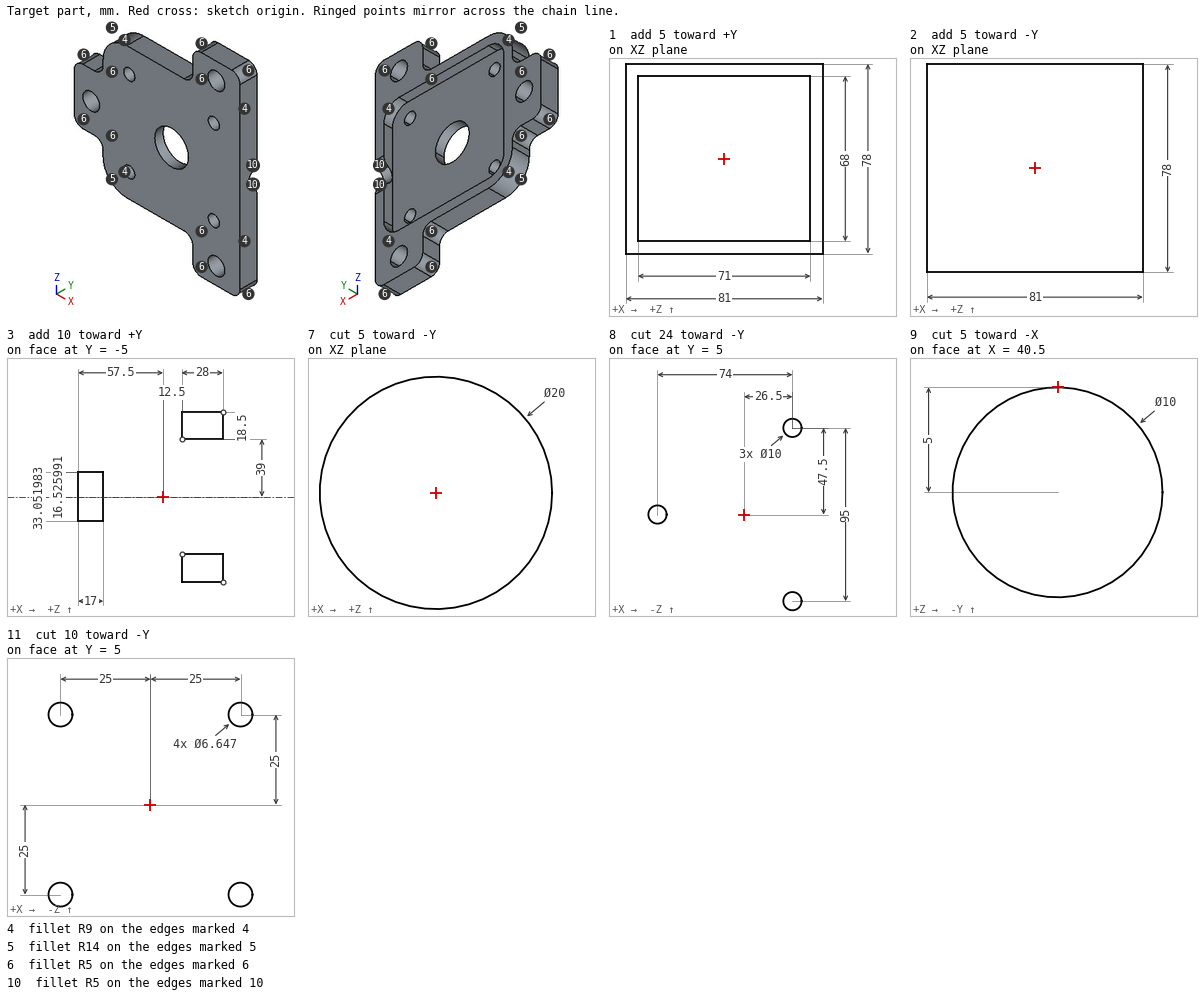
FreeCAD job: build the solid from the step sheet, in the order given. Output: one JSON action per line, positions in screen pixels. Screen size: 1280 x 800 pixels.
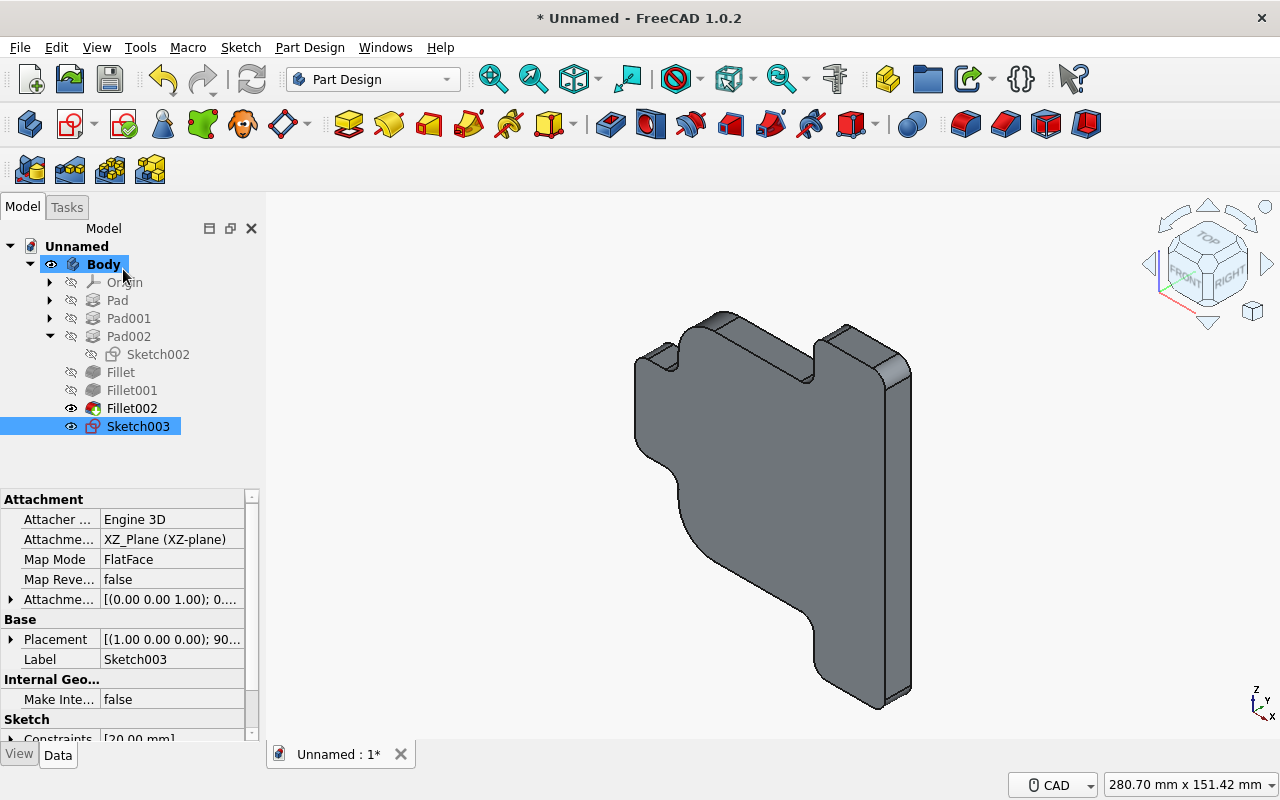
{"action": "left_click", "coordinate": [612, 124]}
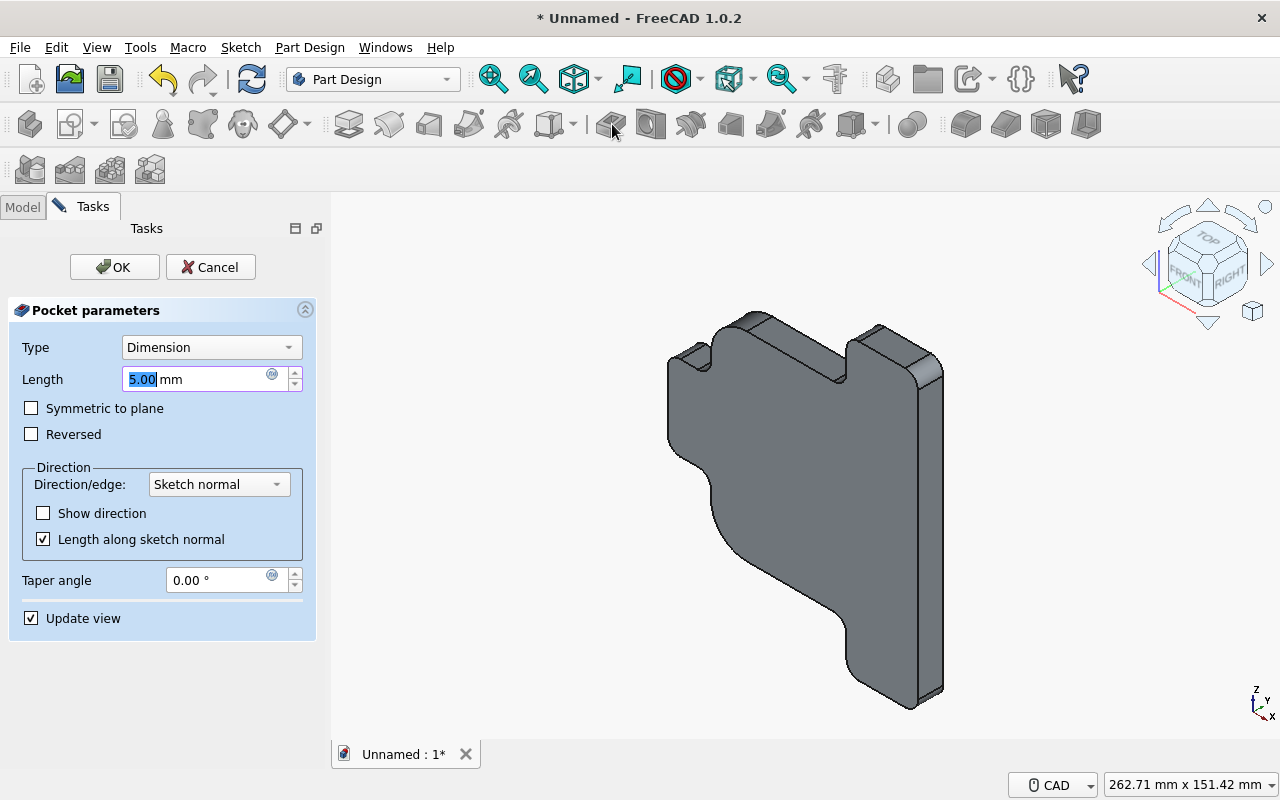
{"action": "type", "text": "5"}
{"action": "key", "text": "Tab"}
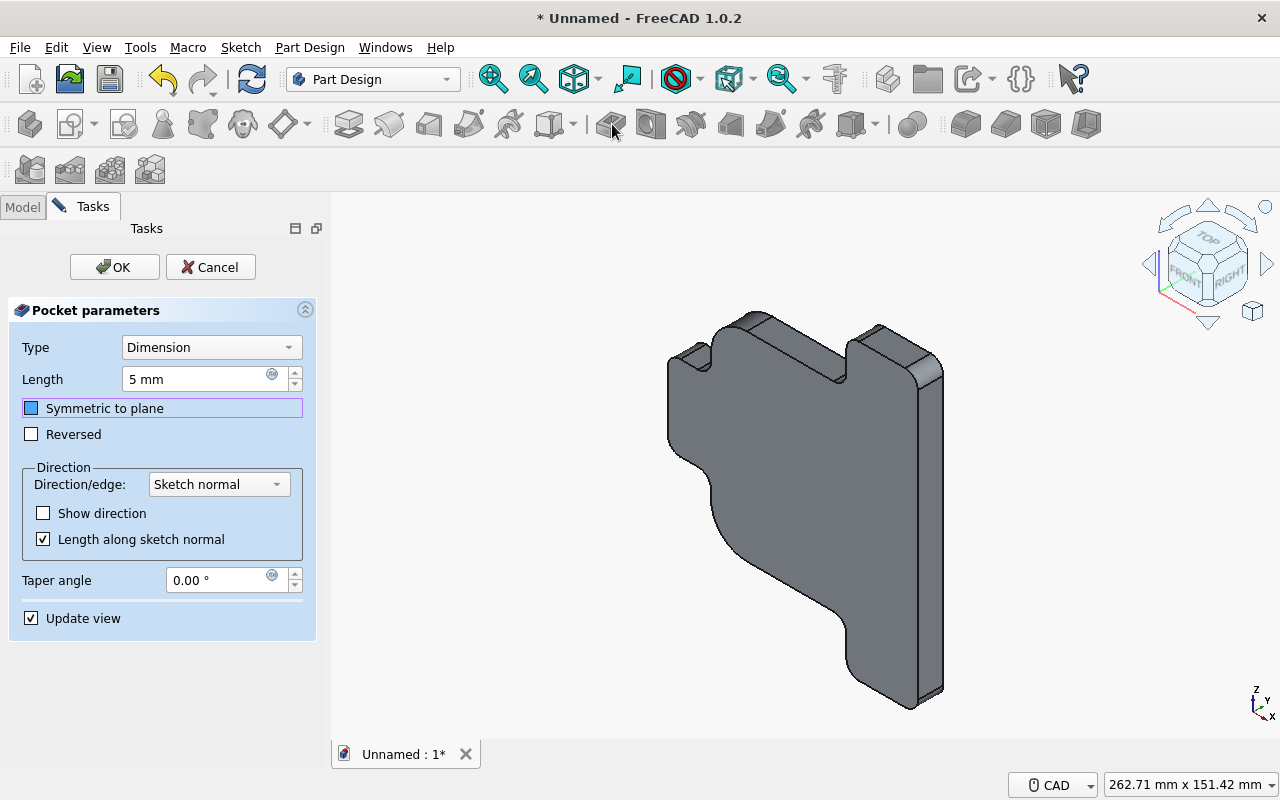
{"action": "left_click", "coordinate": [30, 434]}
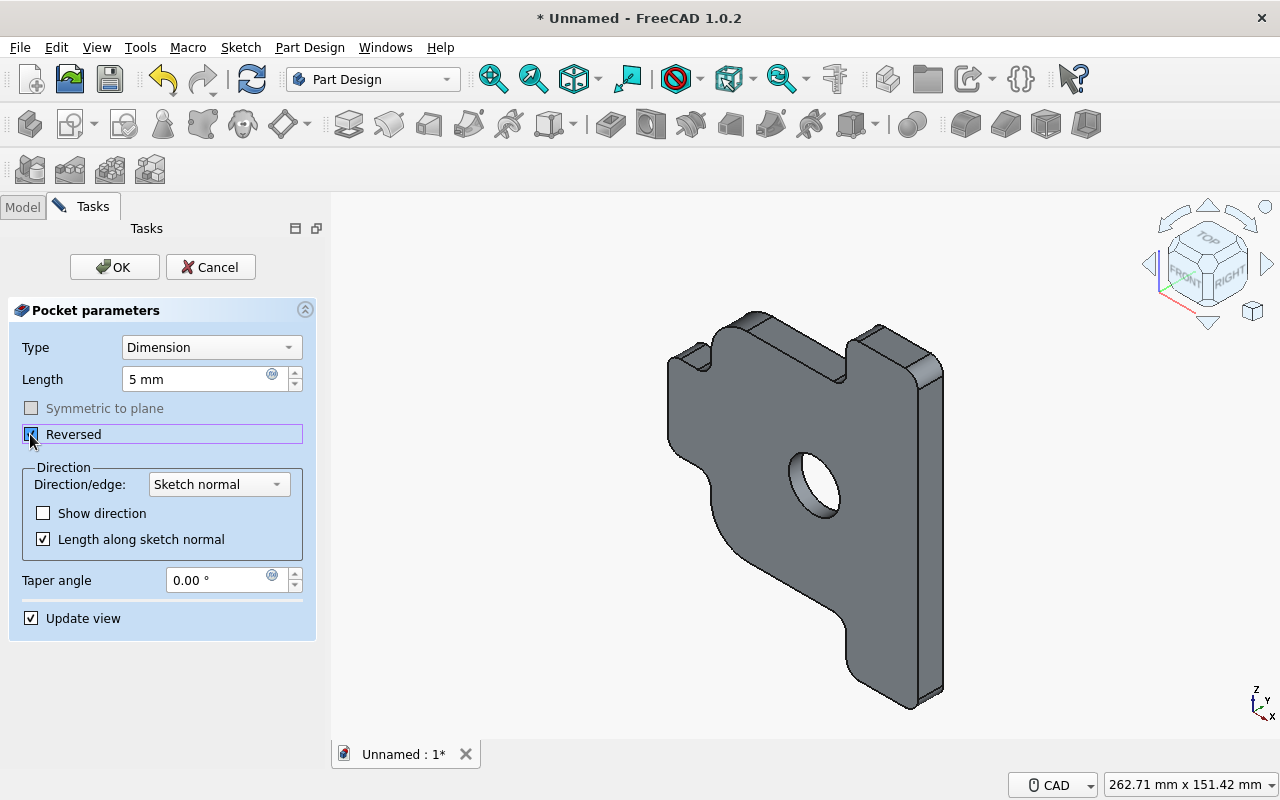
{"action": "left_click", "coordinate": [115, 267]}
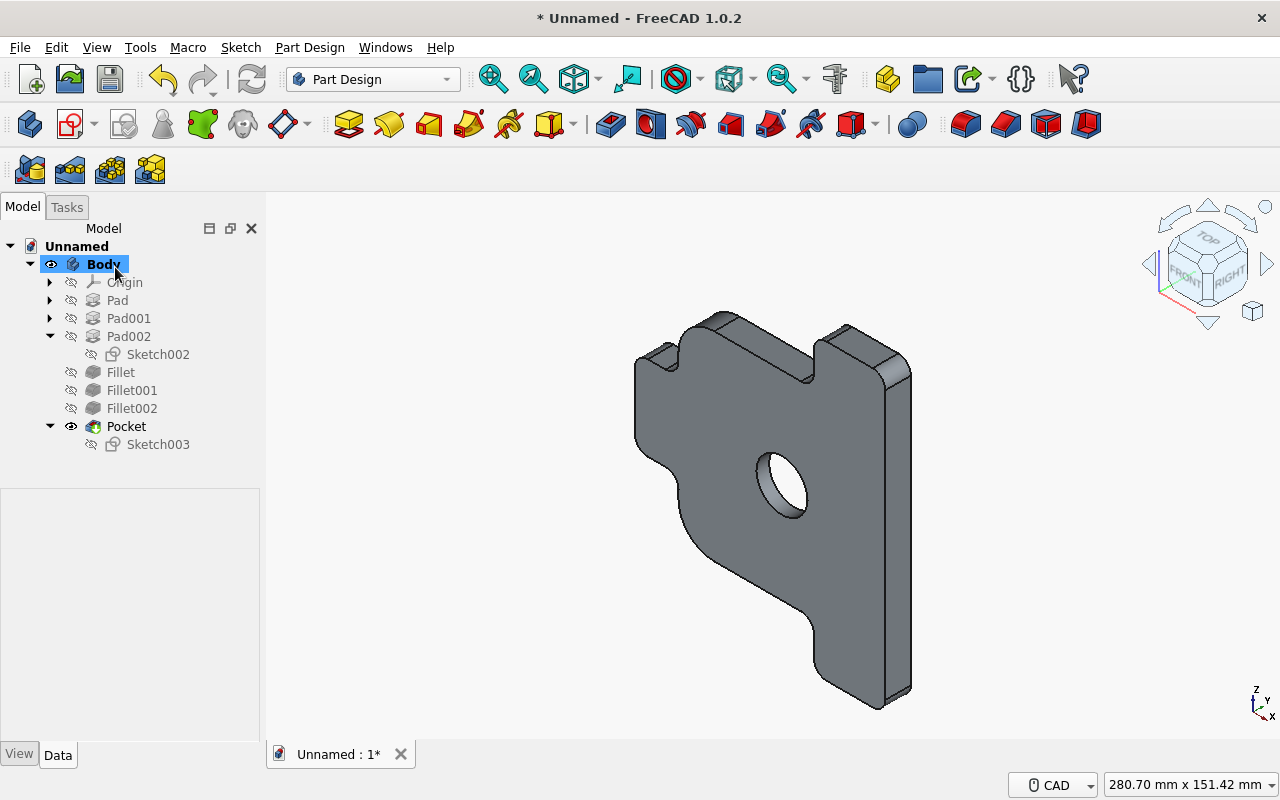
{"action": "key", "text": "4"}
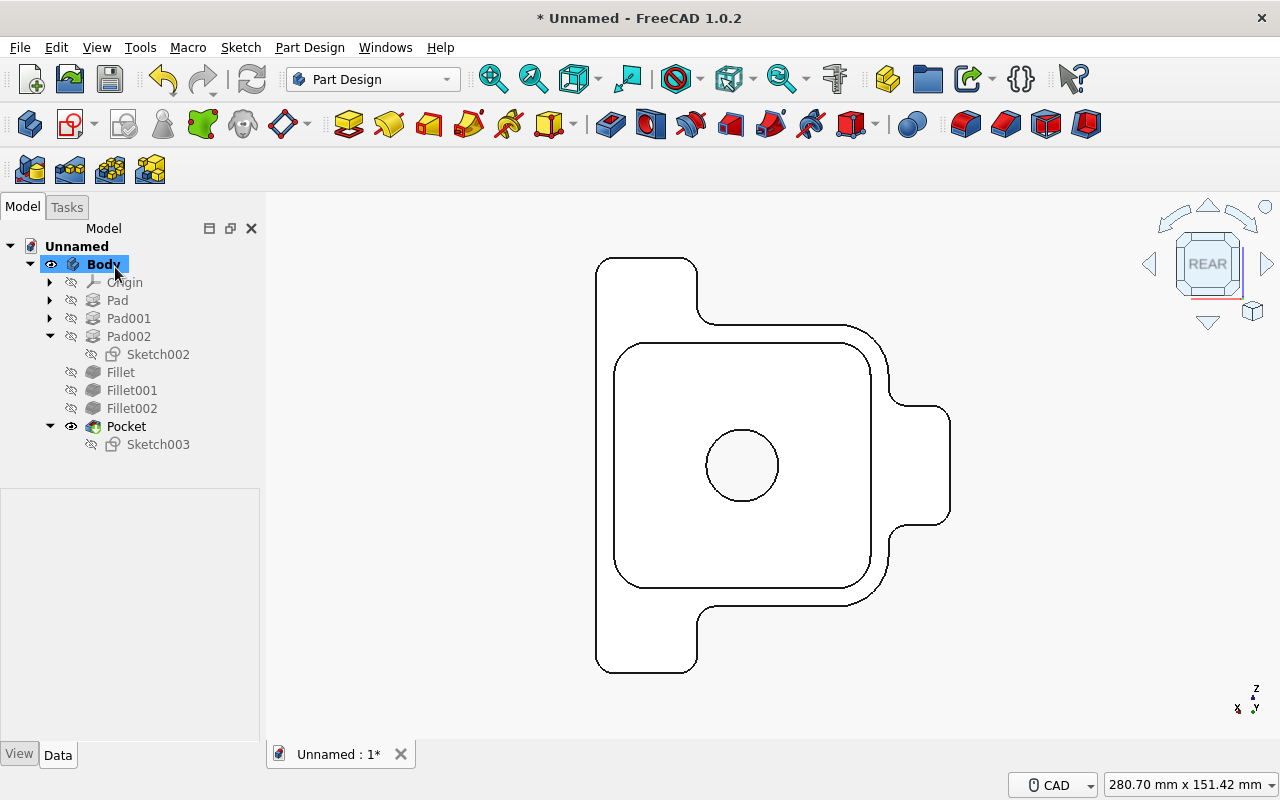
{"action": "left_click", "coordinate": [621, 286]}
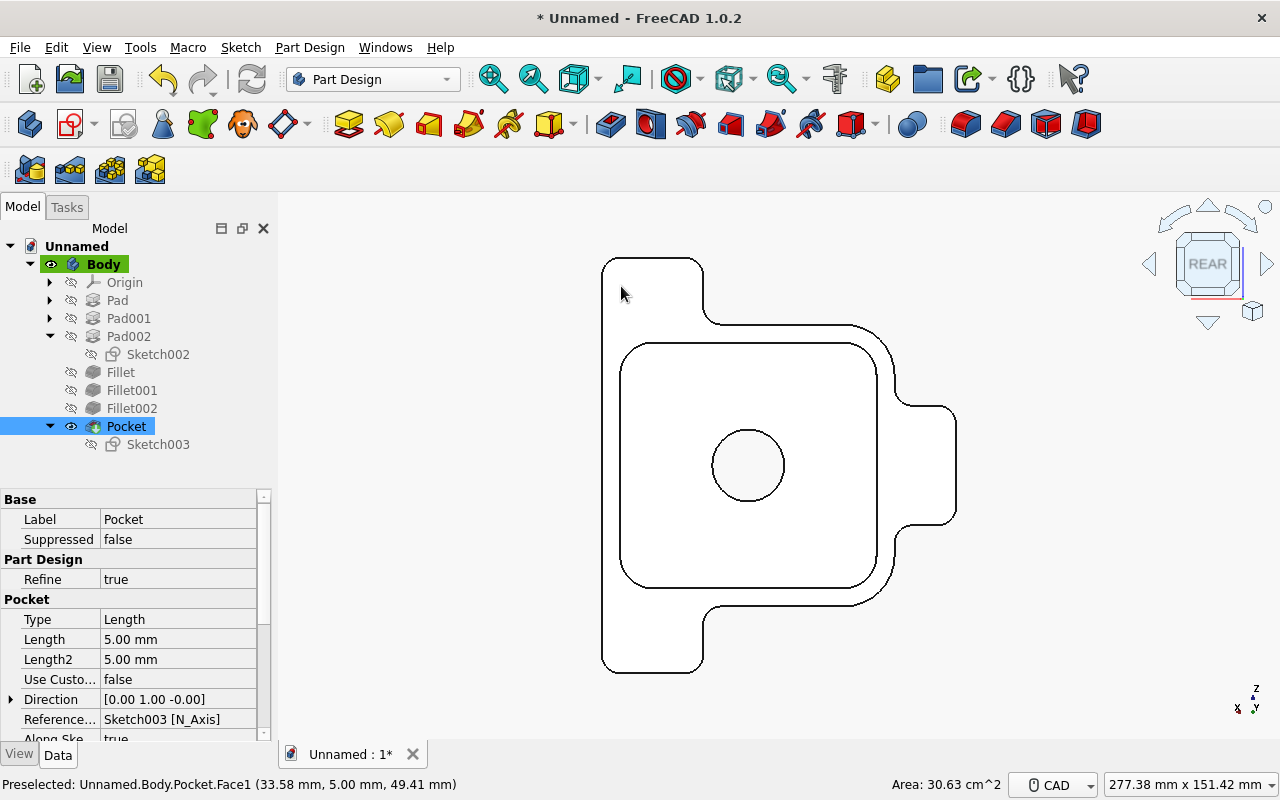
{"action": "left_click", "coordinate": [70, 124]}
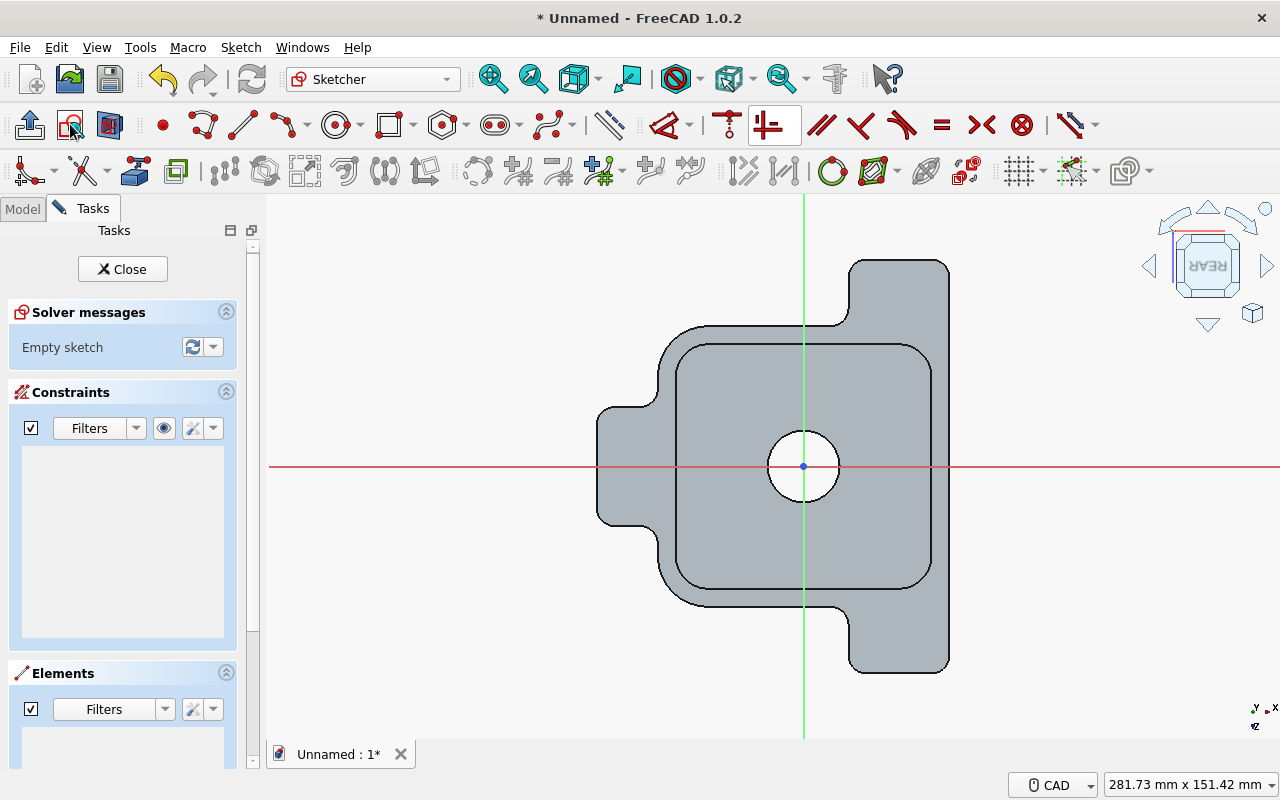
{"action": "key", "text": "g c"}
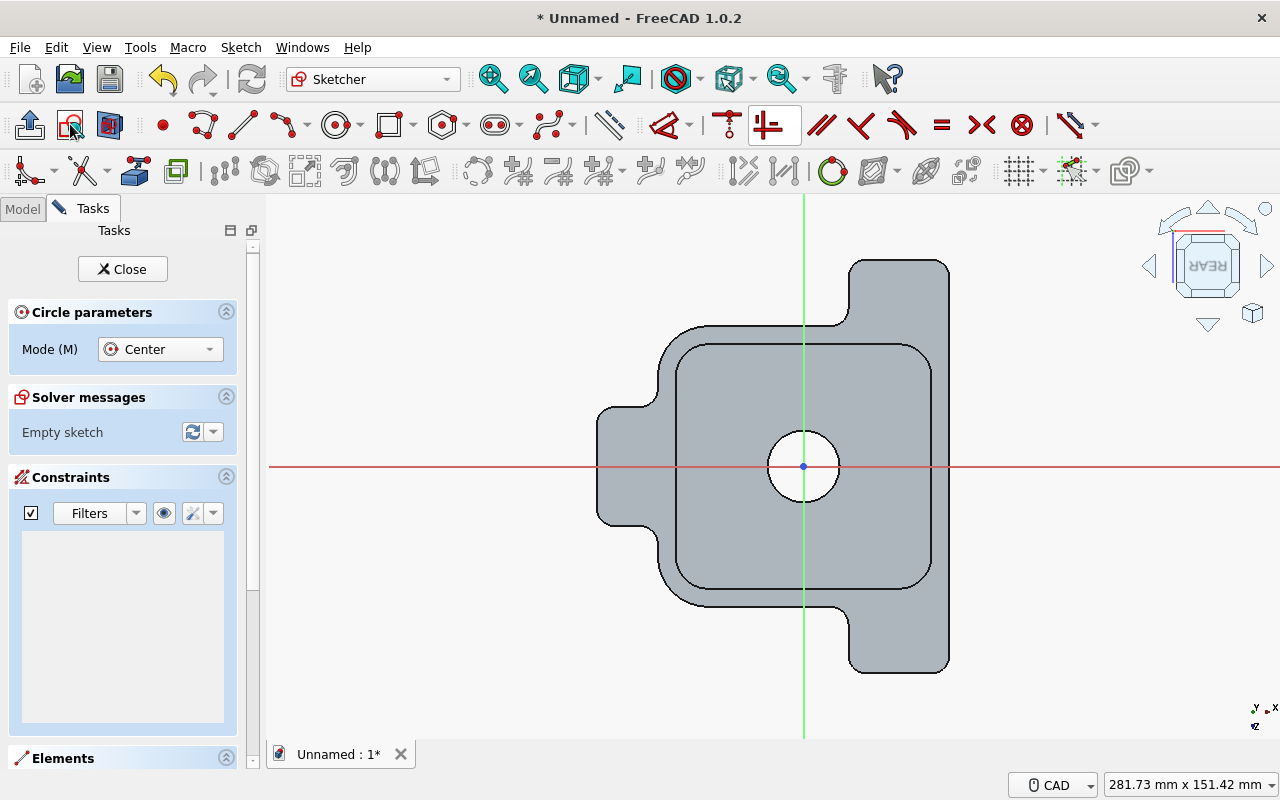
{"action": "scroll", "coordinate": [899, 296], "scroll_direction": "up", "scroll_amount": 2}